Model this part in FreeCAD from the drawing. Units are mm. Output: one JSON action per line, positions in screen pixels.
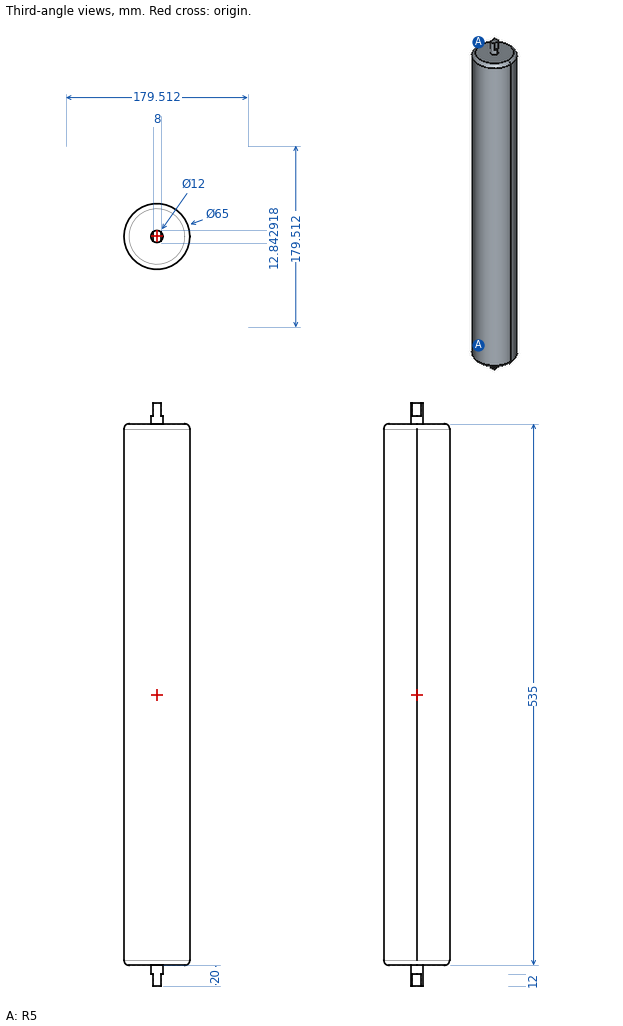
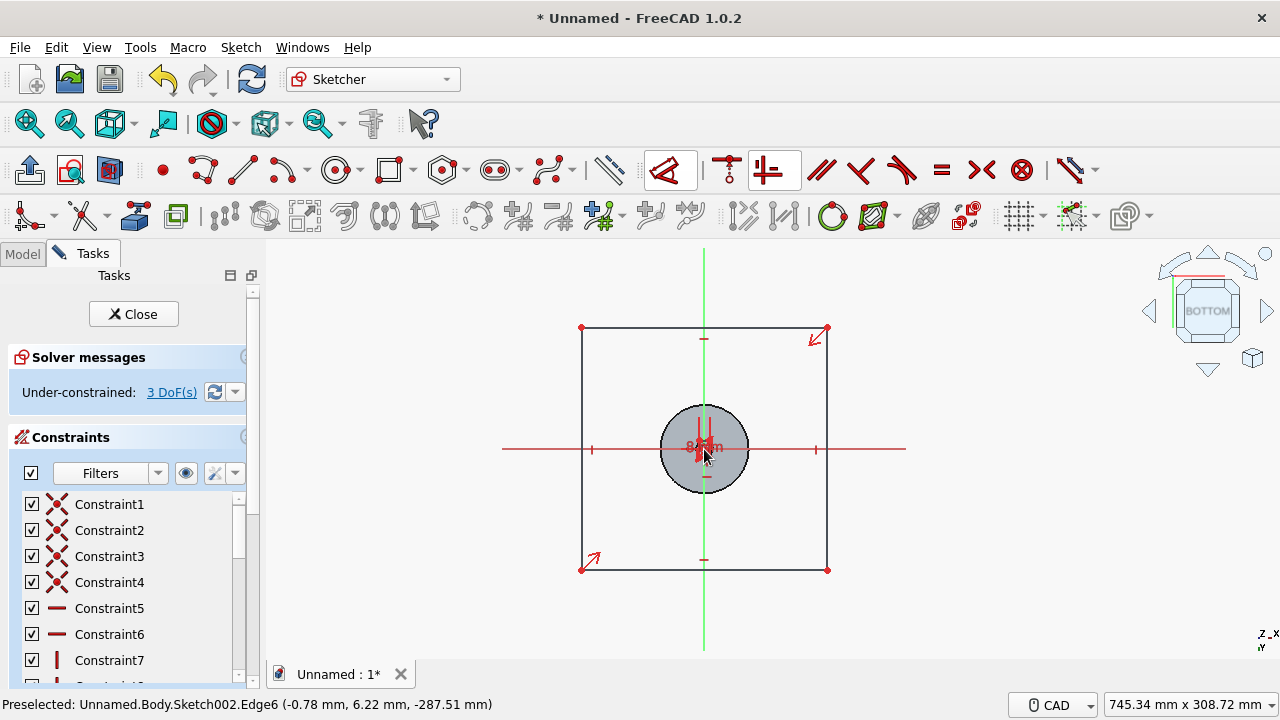
{"action": "left_click", "coordinate": [655, 570]}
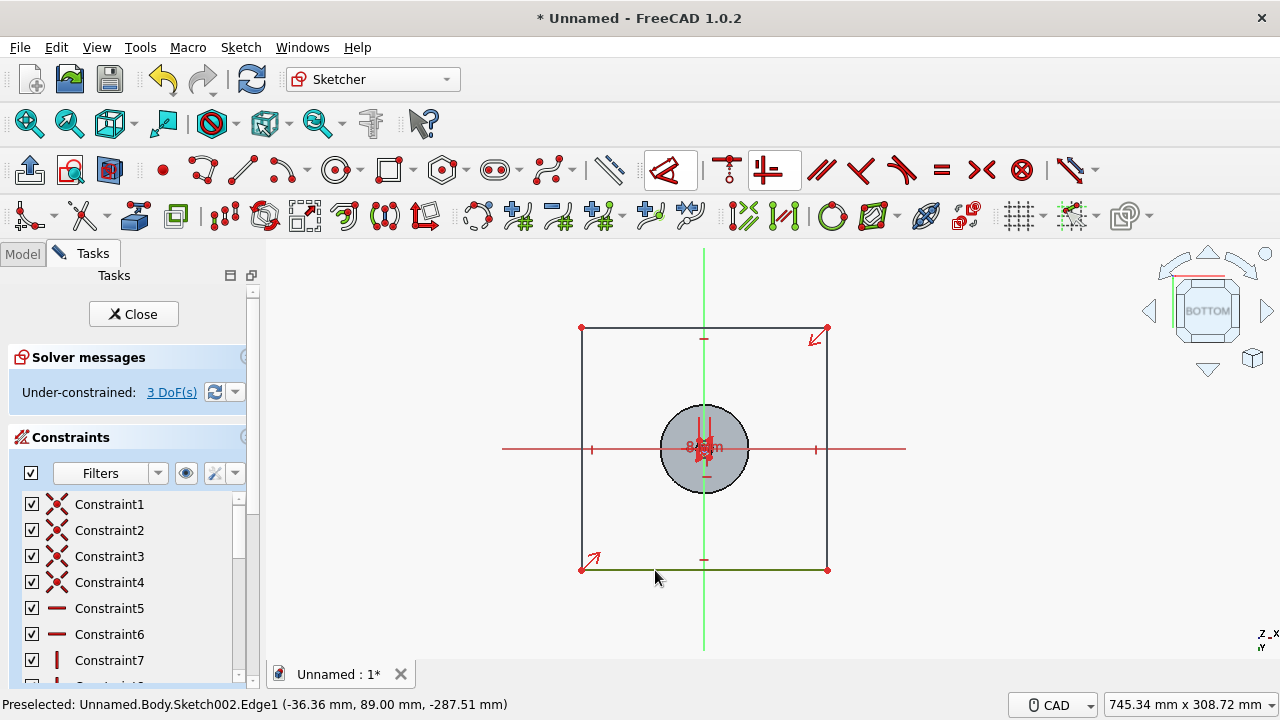
{"action": "left_click", "coordinate": [692, 170]}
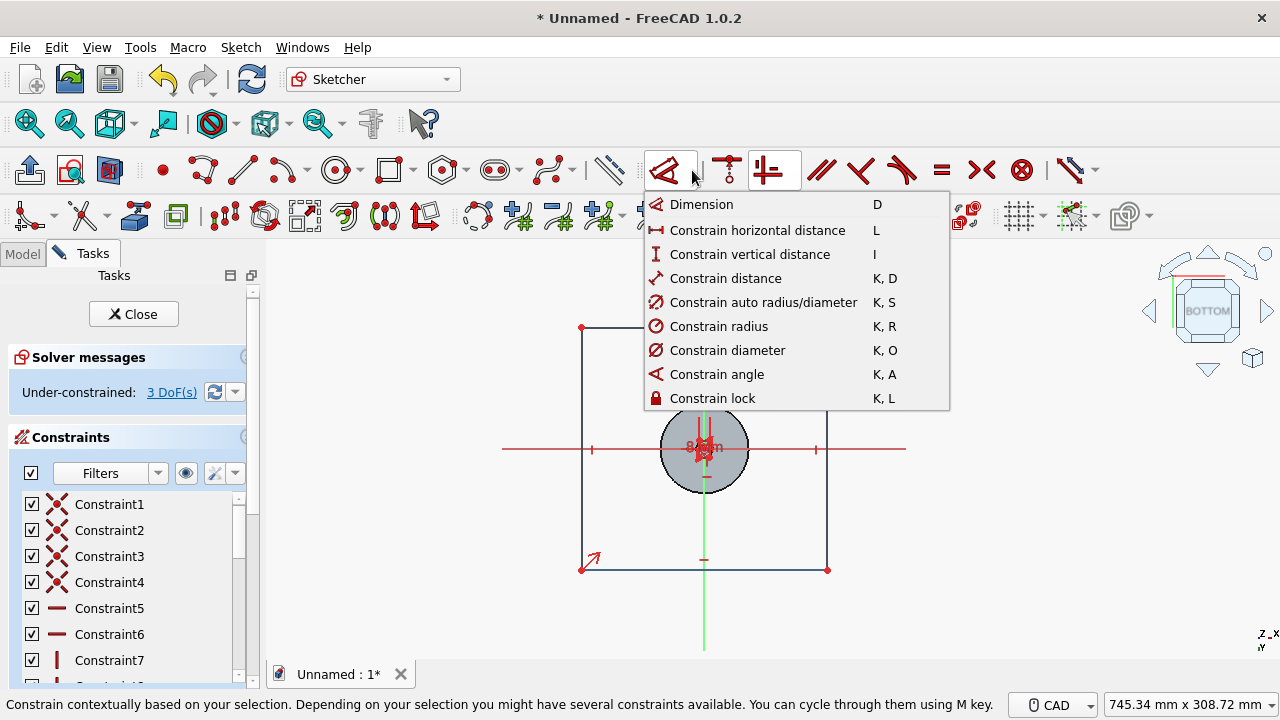
{"action": "left_click", "coordinate": [797, 230]}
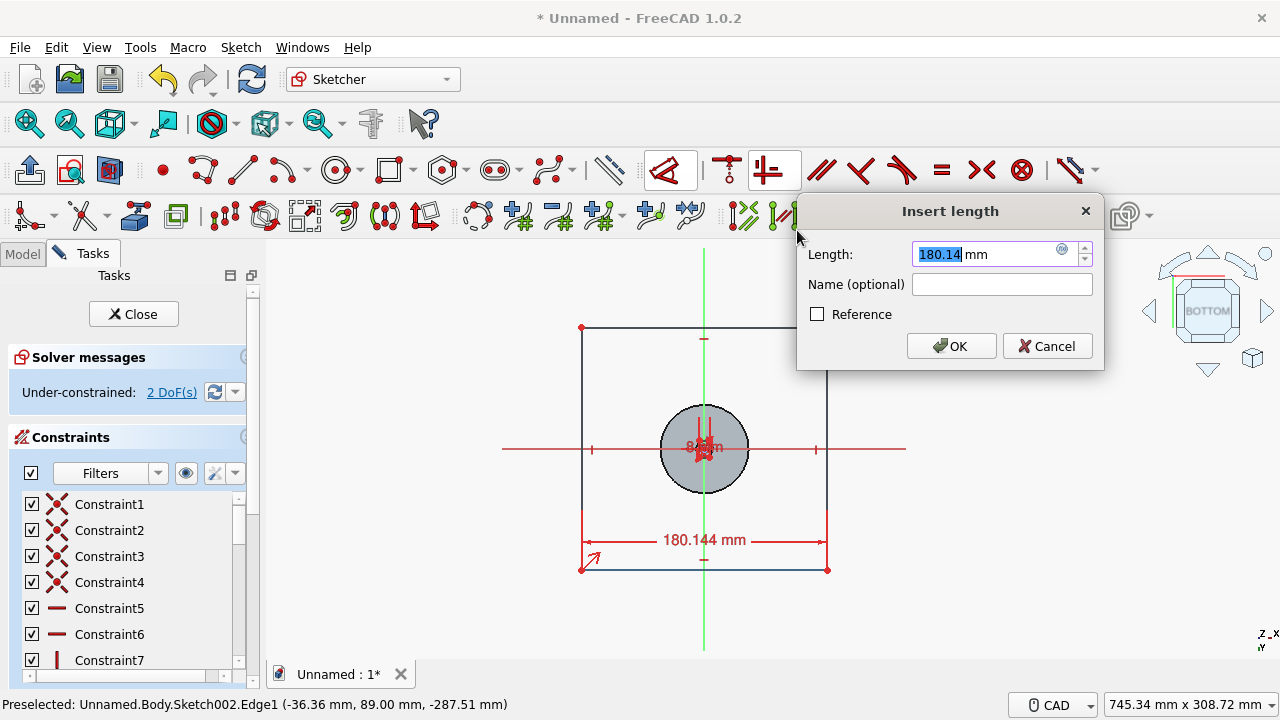
{"action": "type", "text": "179.512"}
{"action": "key", "text": "Return"}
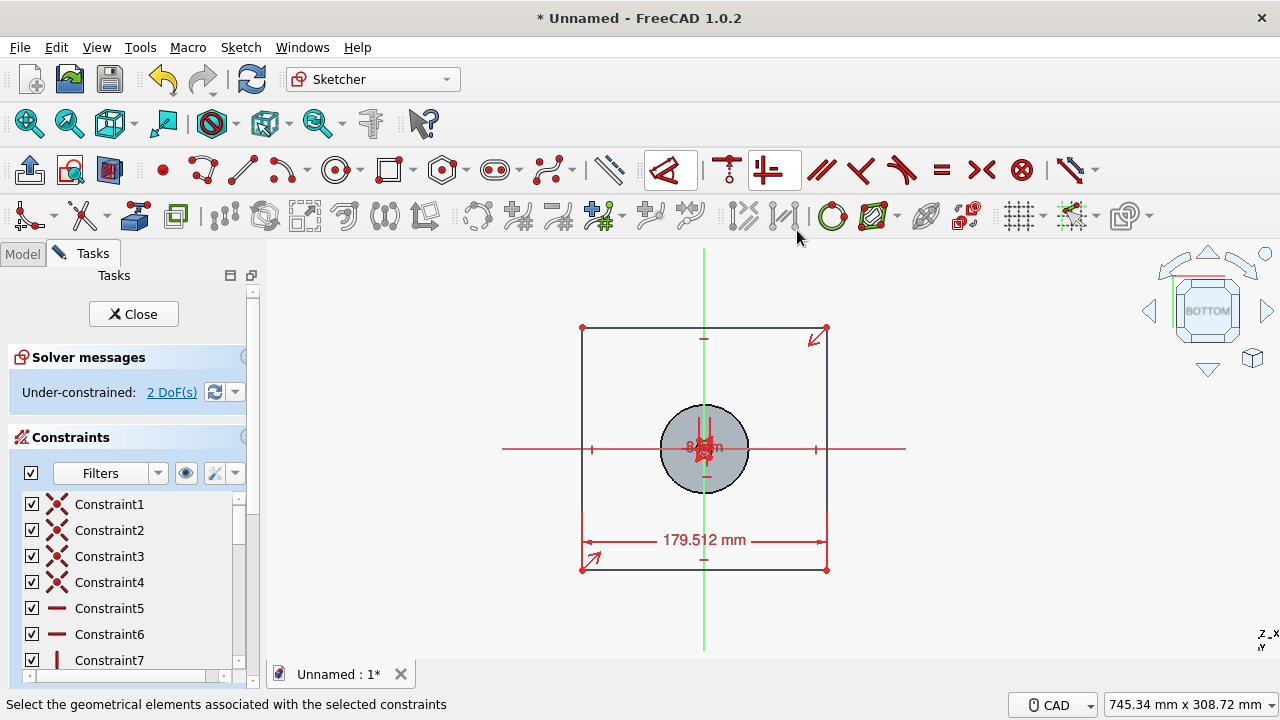
{"action": "left_click", "coordinate": [827, 498]}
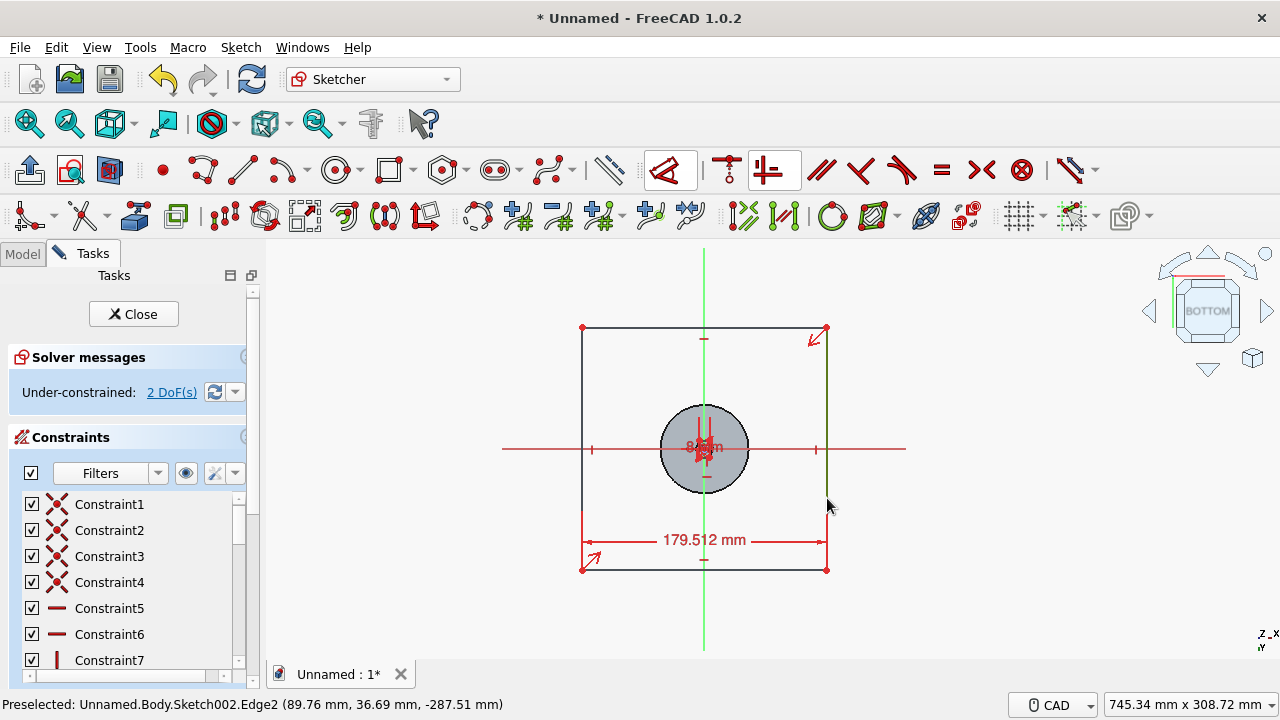
{"action": "key", "text": "i"}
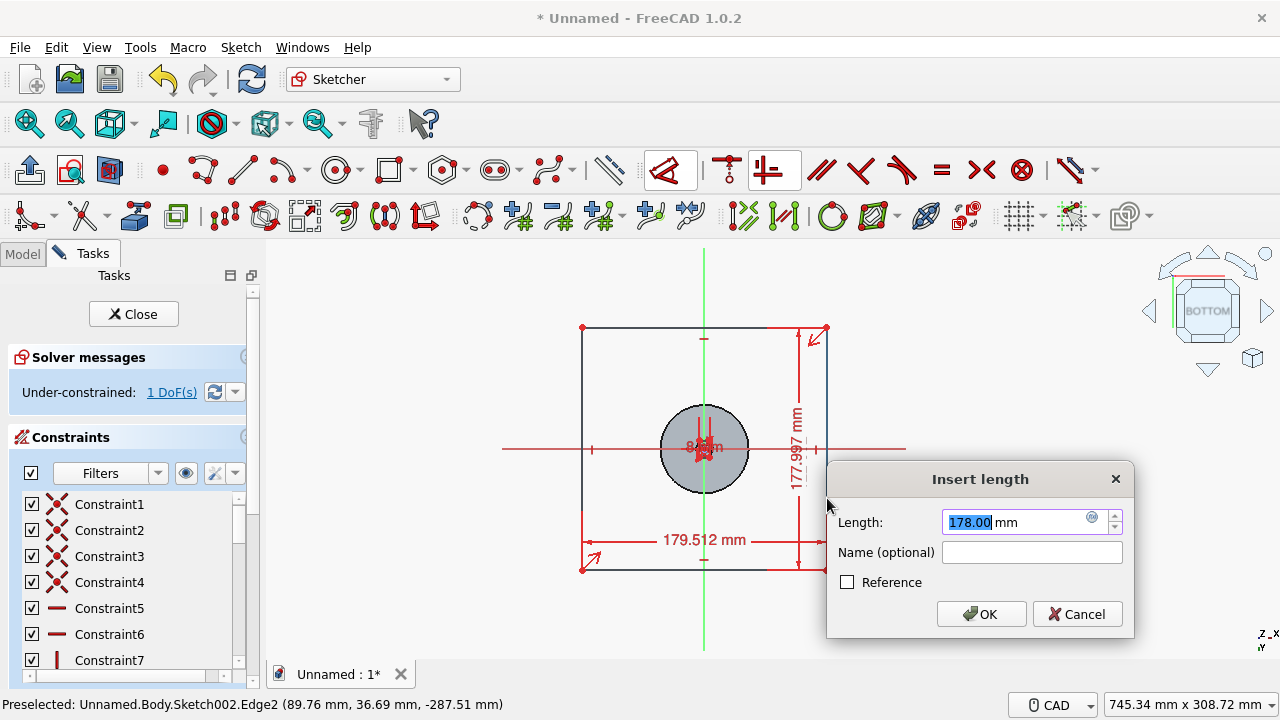
{"action": "type", "text": "179.512"}
{"action": "key", "text": "Return"}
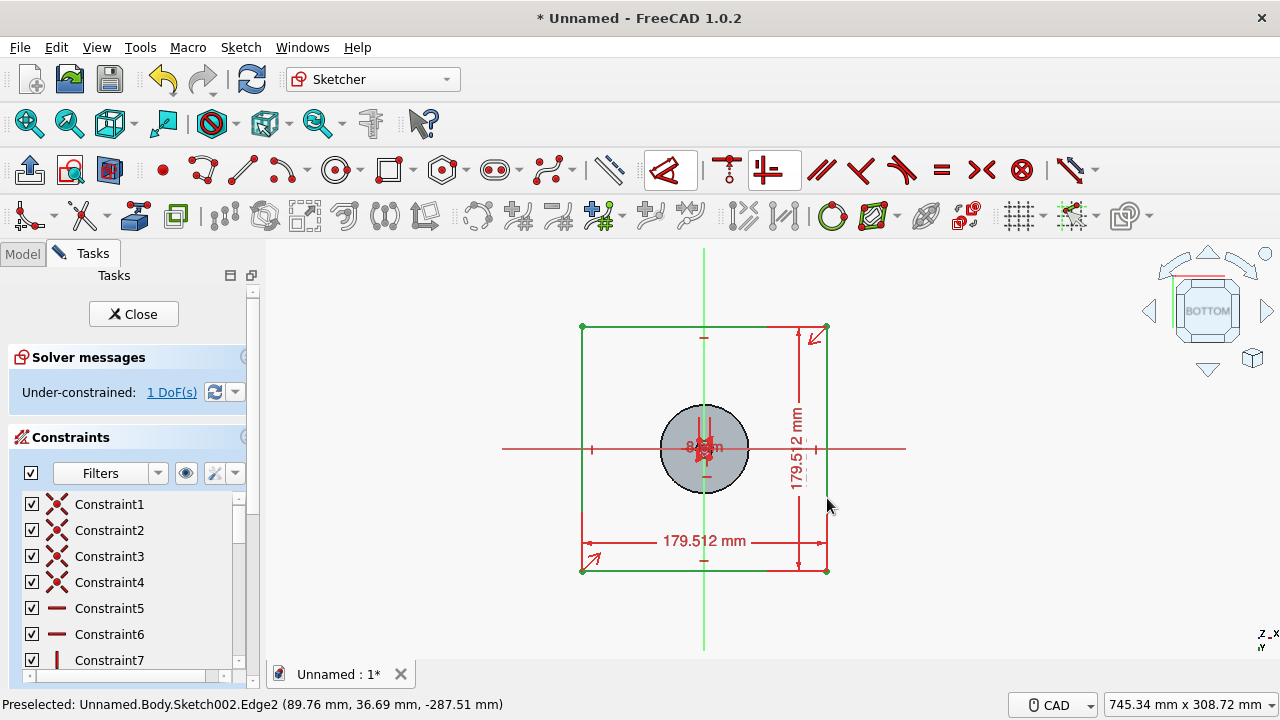
{"action": "scroll", "coordinate": [710, 451], "scroll_direction": "up", "scroll_amount": 5}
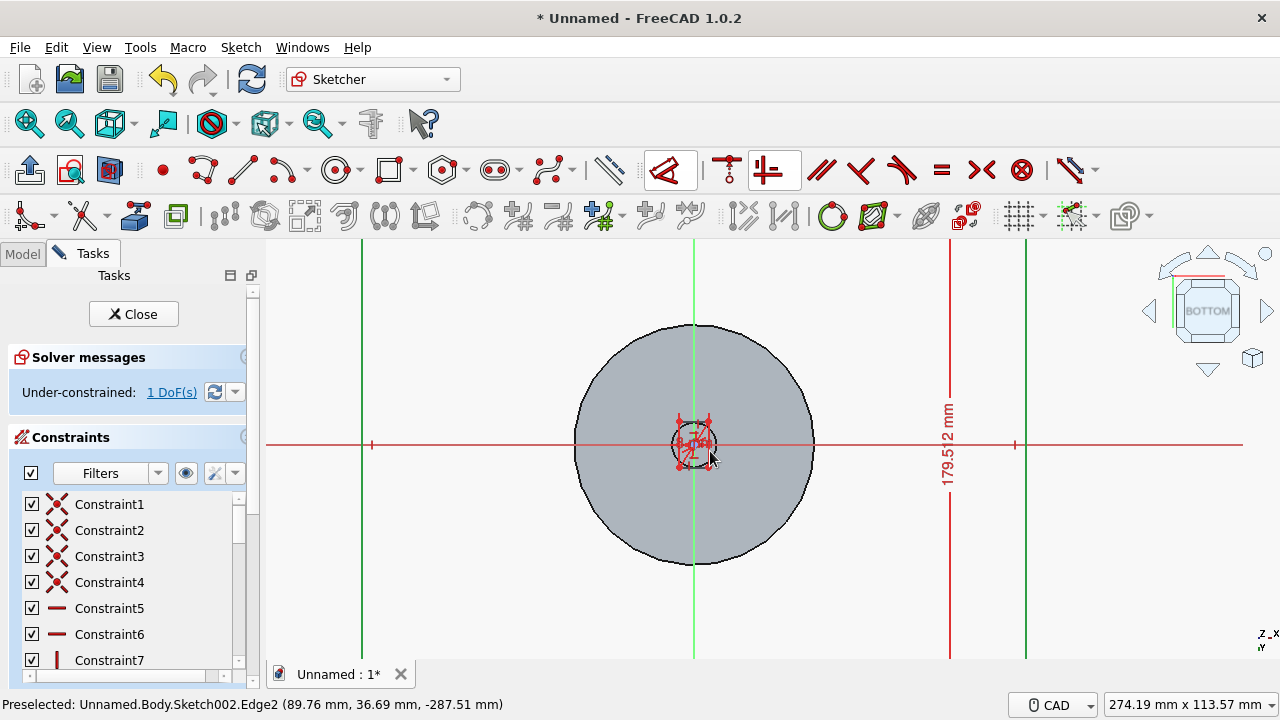
{"action": "left_click", "coordinate": [709, 454]}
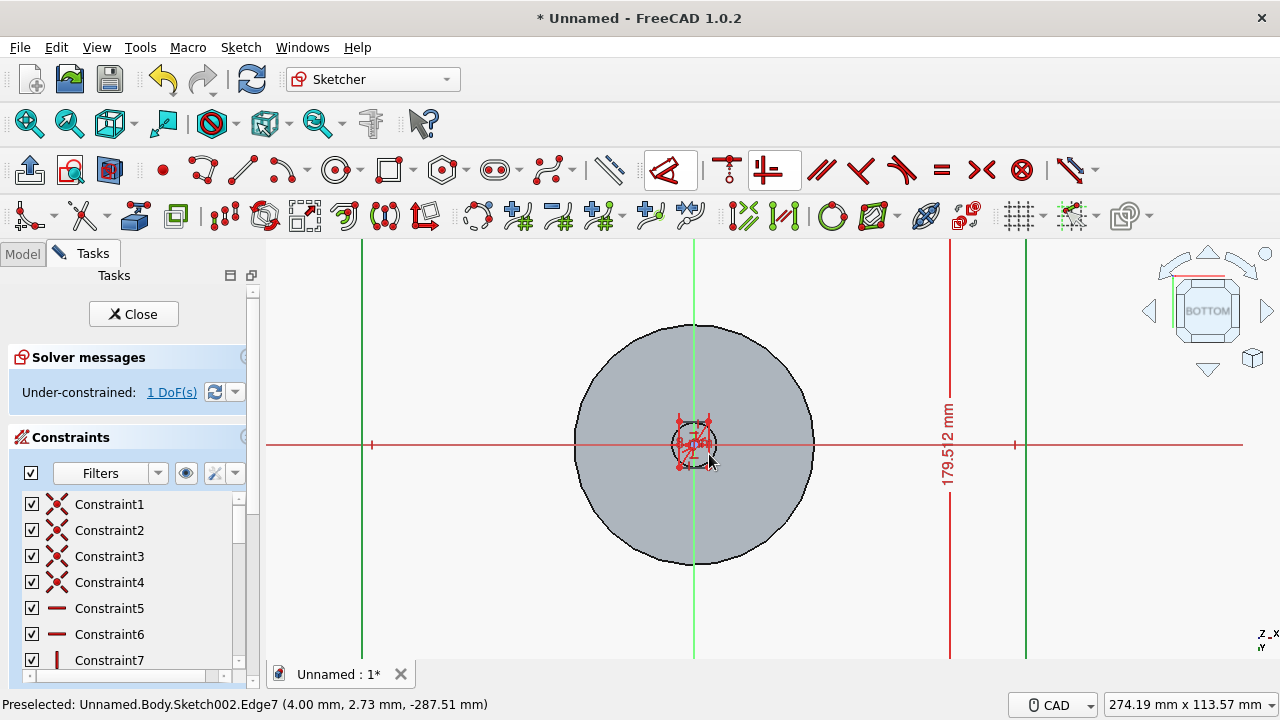
{"action": "key", "text": "i"}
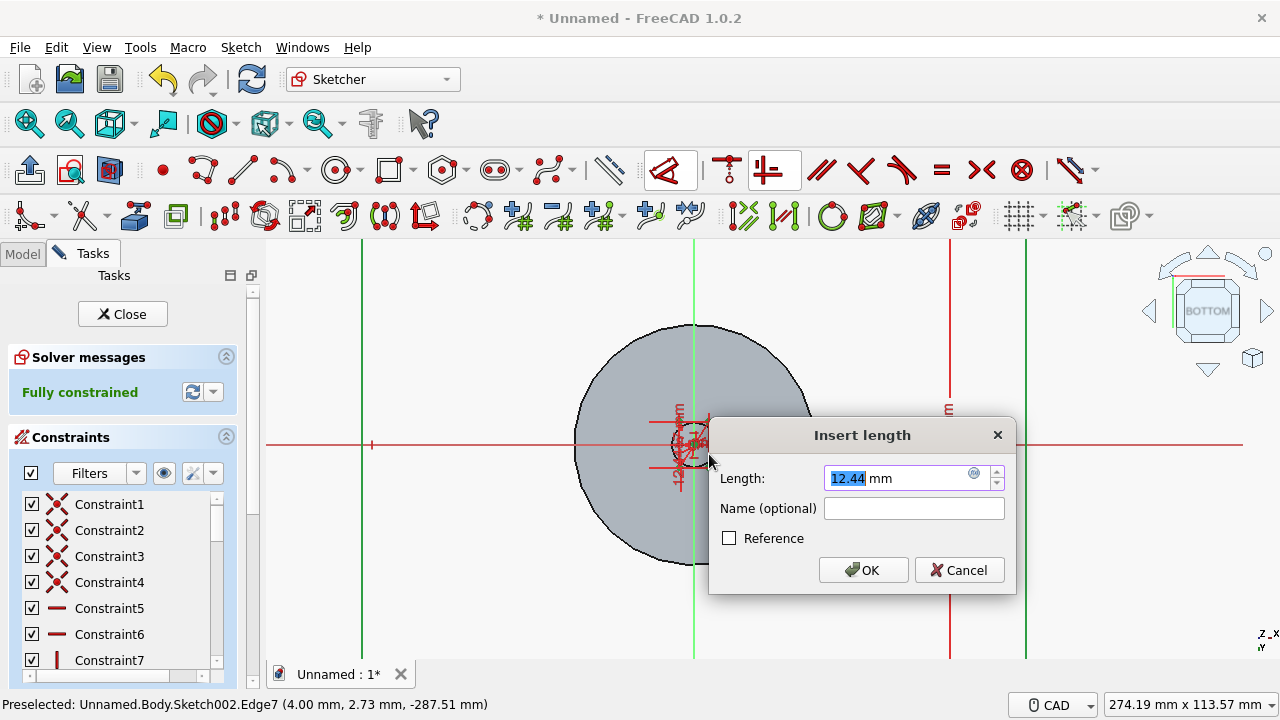
{"action": "type", "text": "12.842918"}
{"action": "key", "text": "Return"}